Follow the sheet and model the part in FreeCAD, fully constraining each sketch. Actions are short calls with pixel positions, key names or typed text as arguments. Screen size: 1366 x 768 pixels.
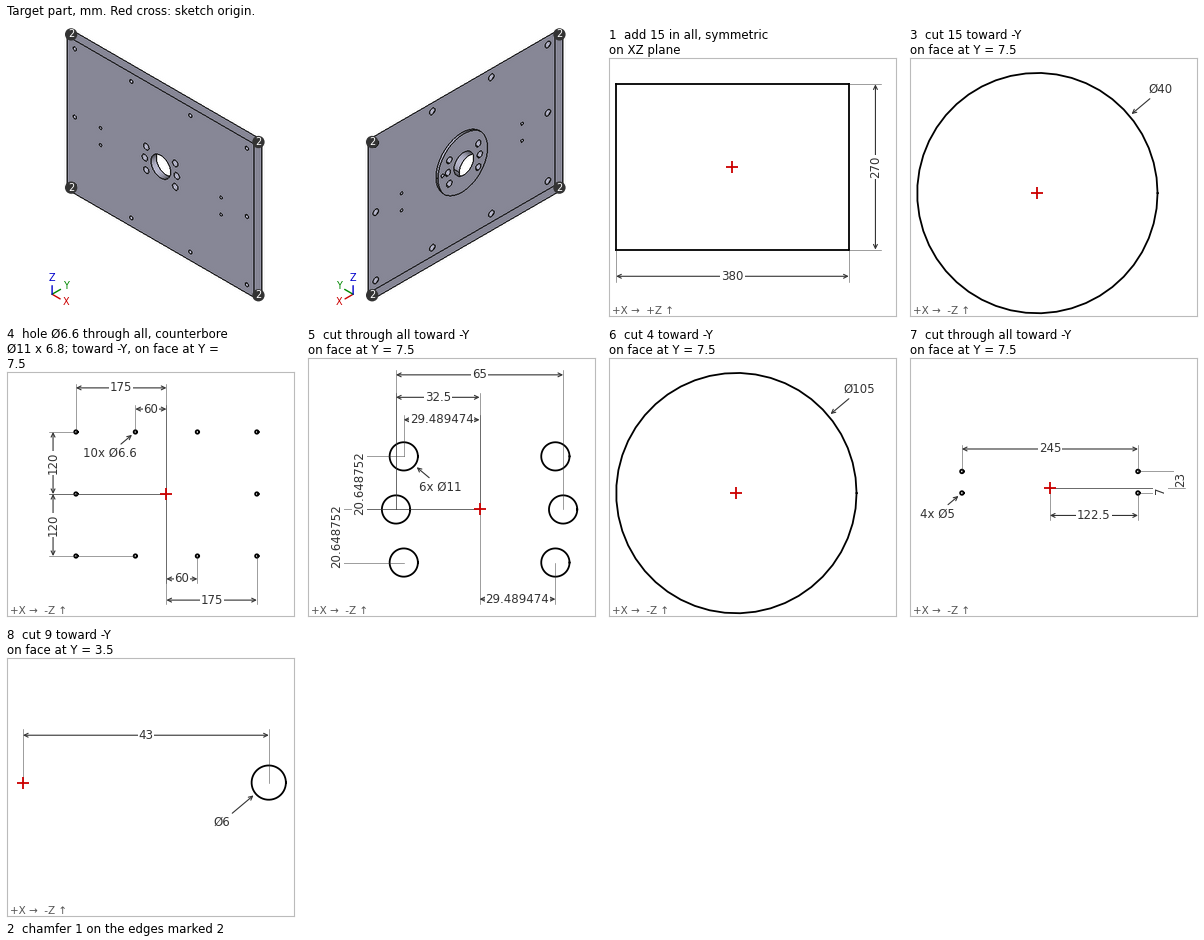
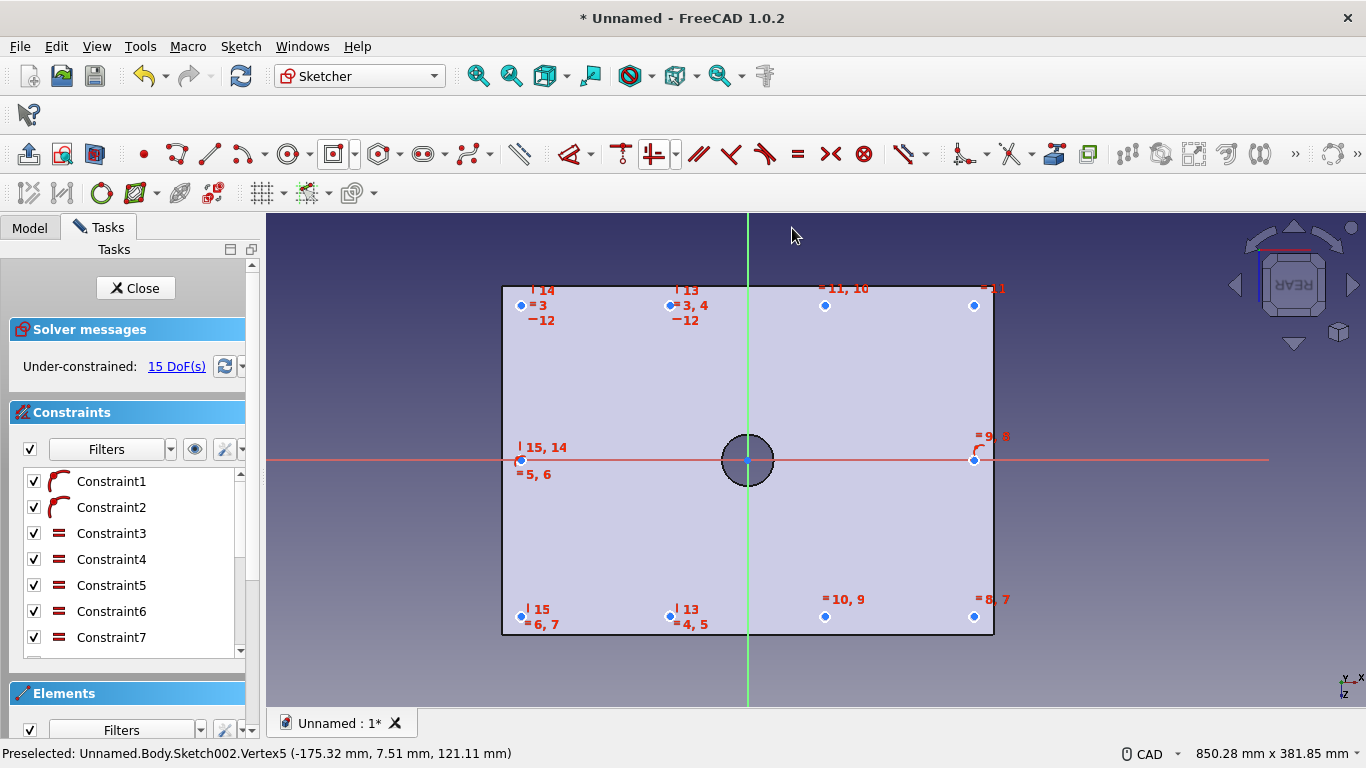
click(670, 616)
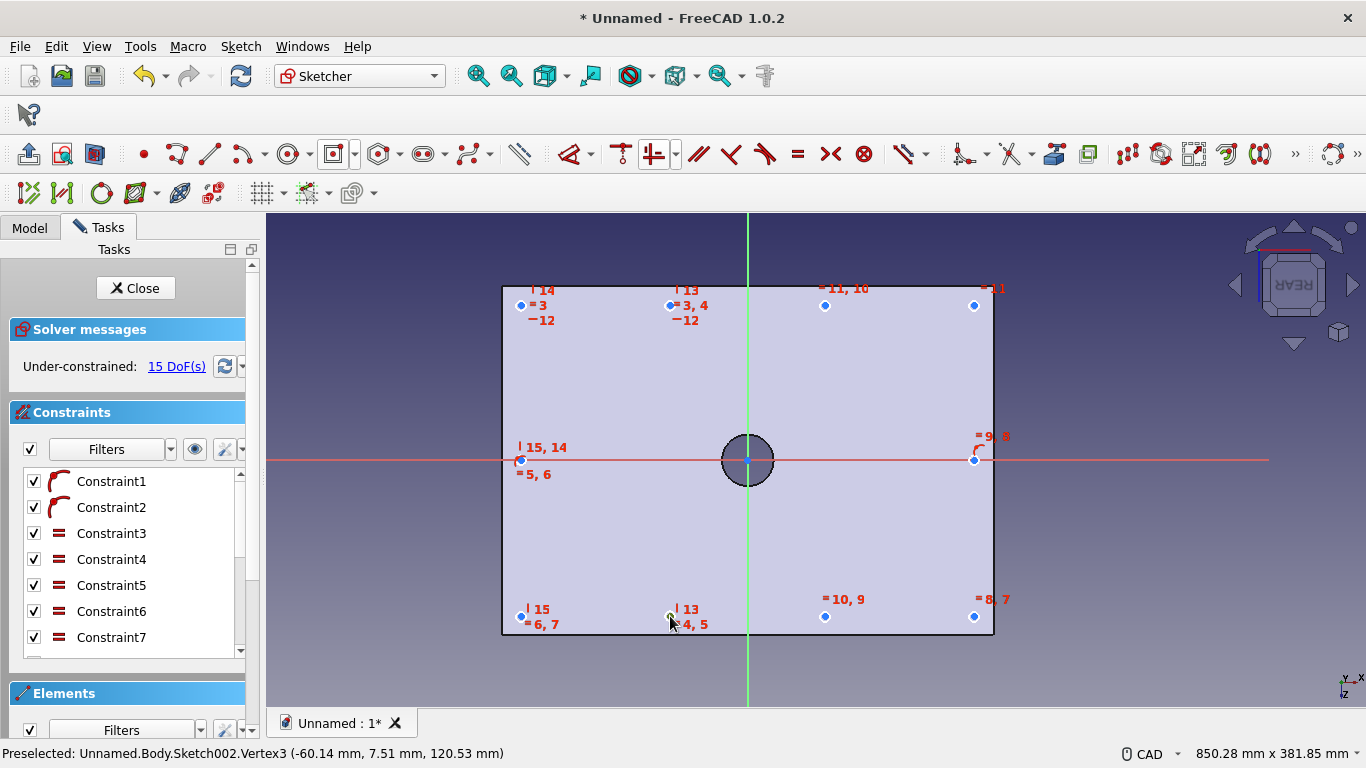
click(521, 617)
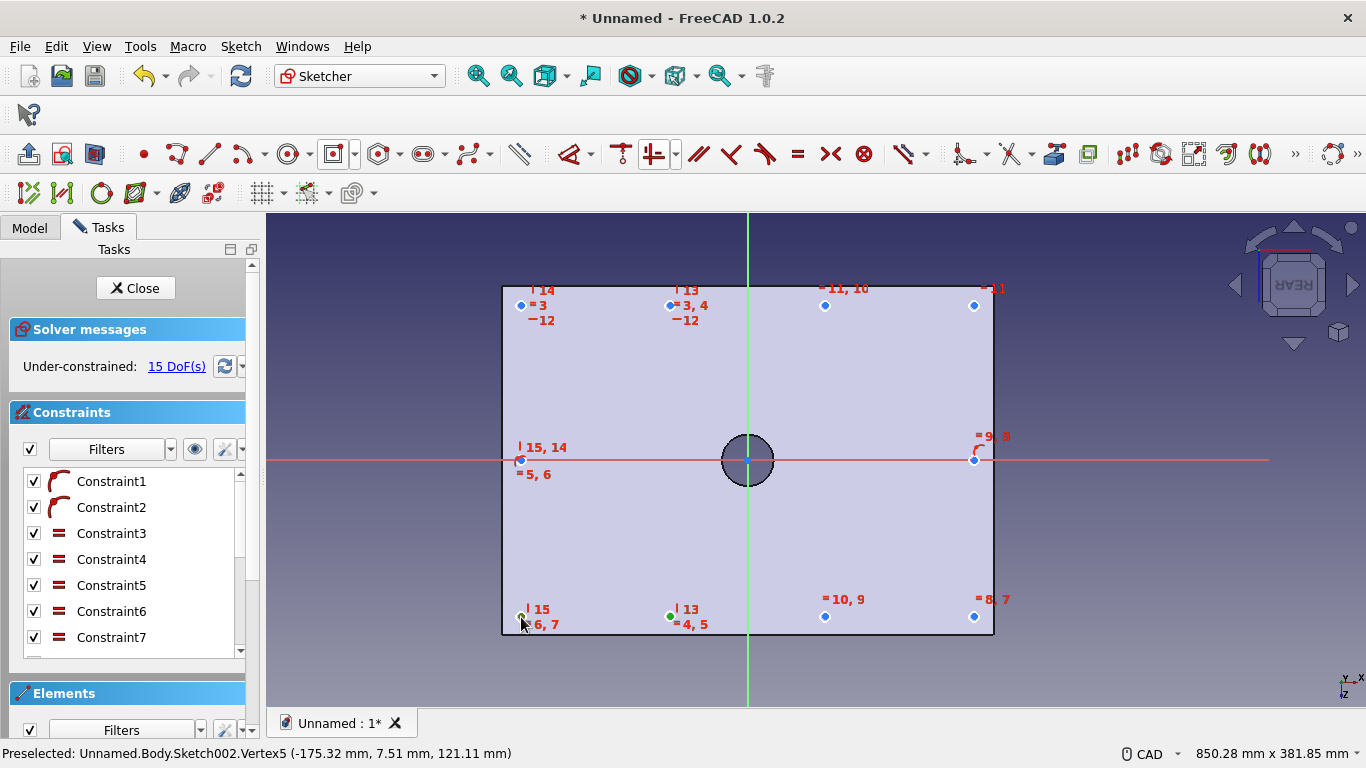
click(676, 154)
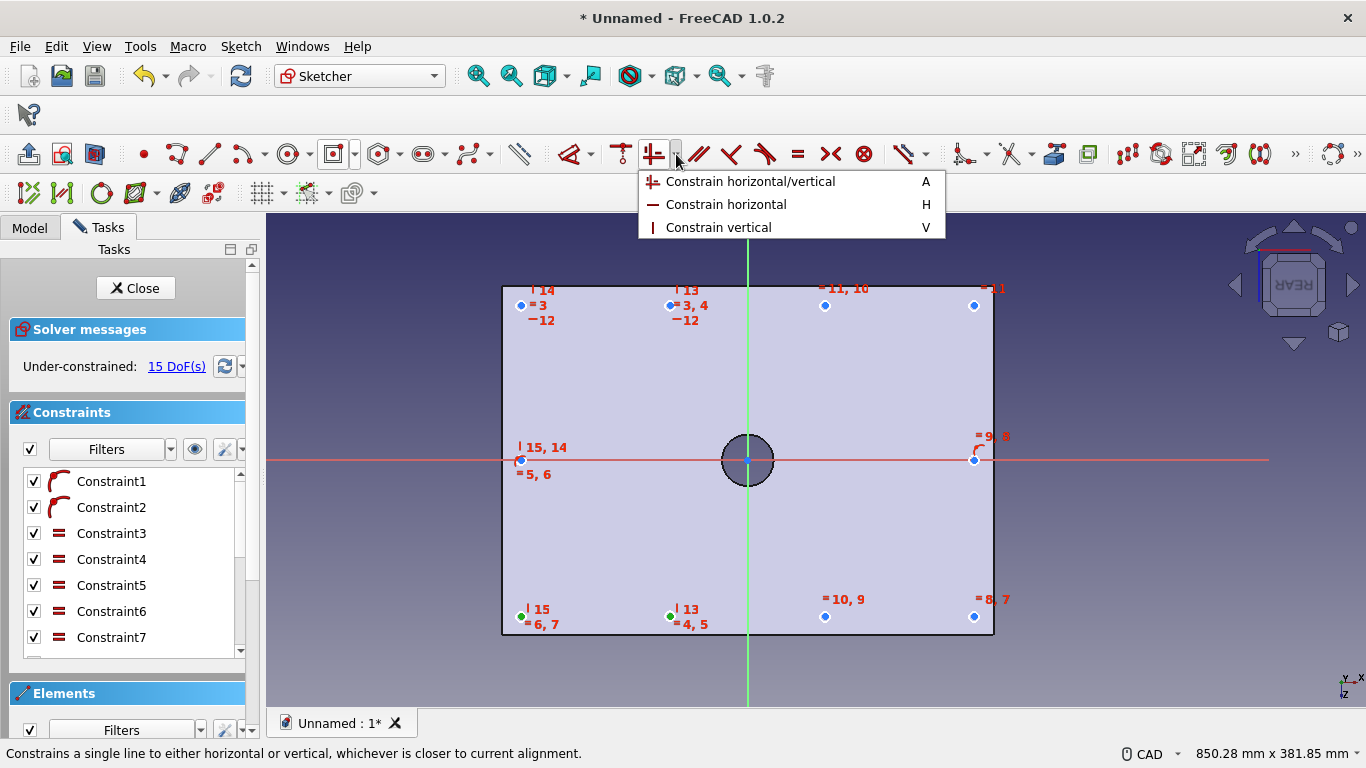
click(792, 204)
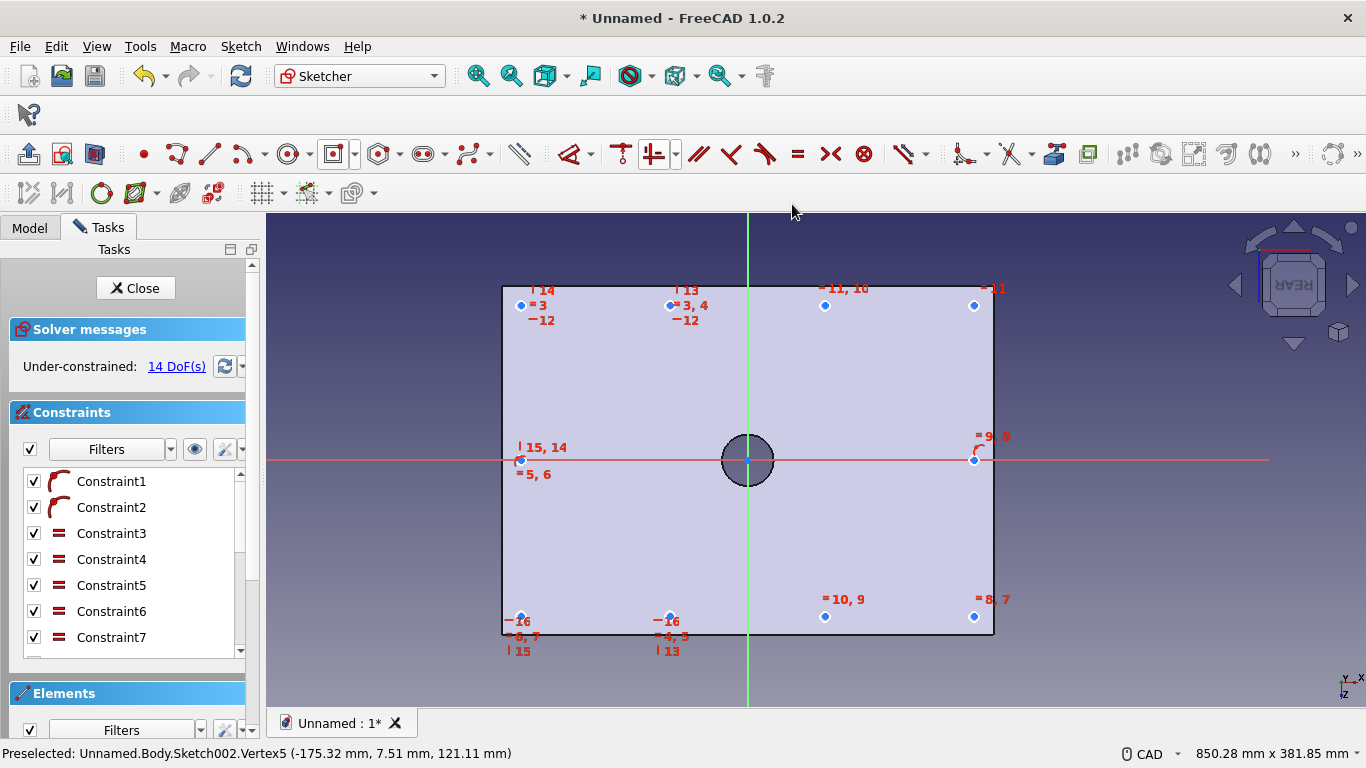
click(670, 616)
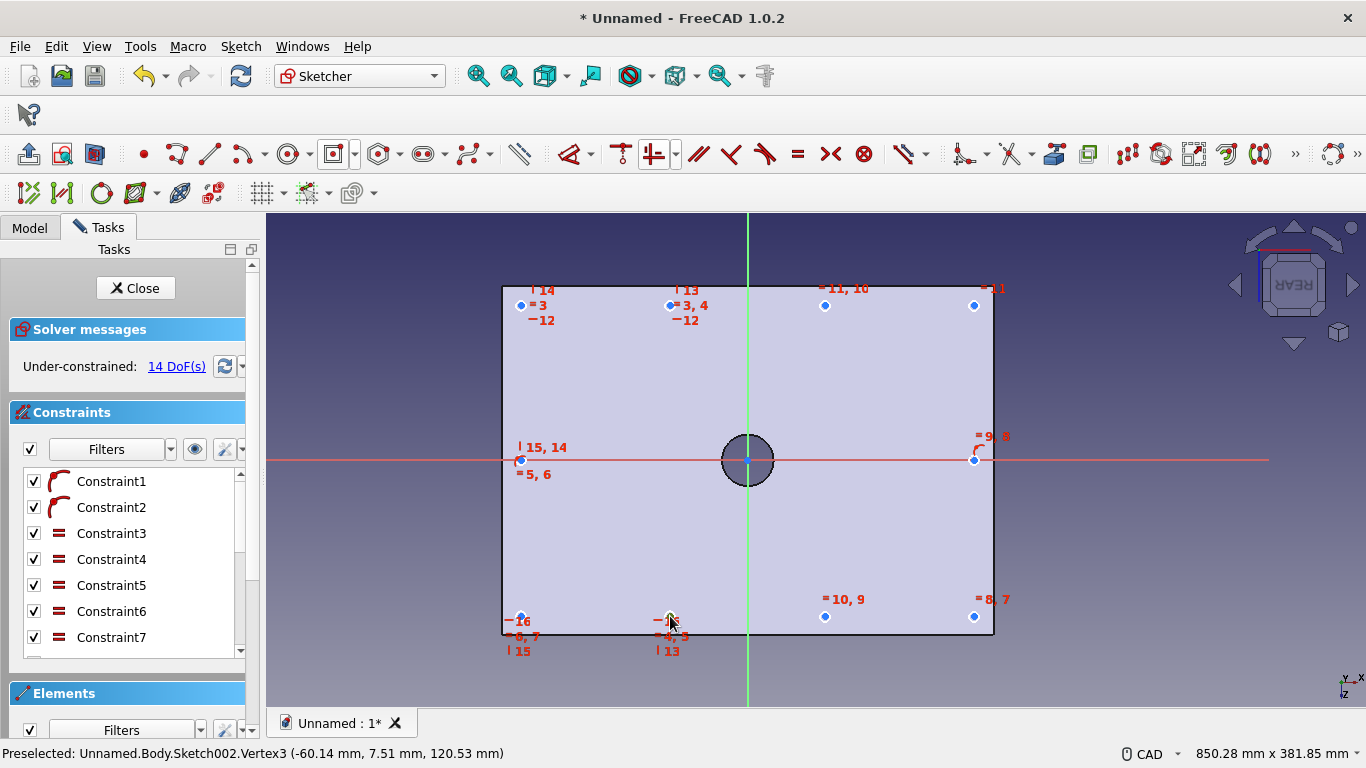
click(974, 617)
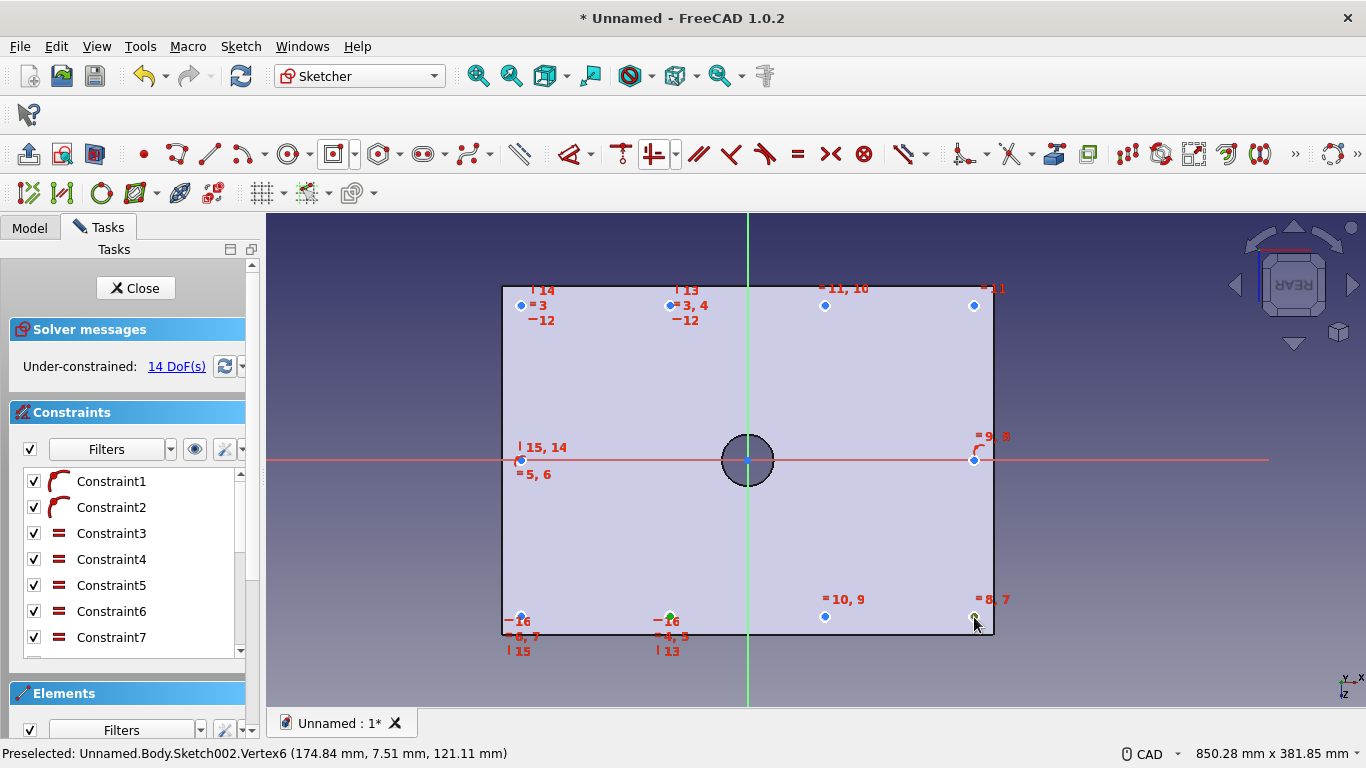
key(h)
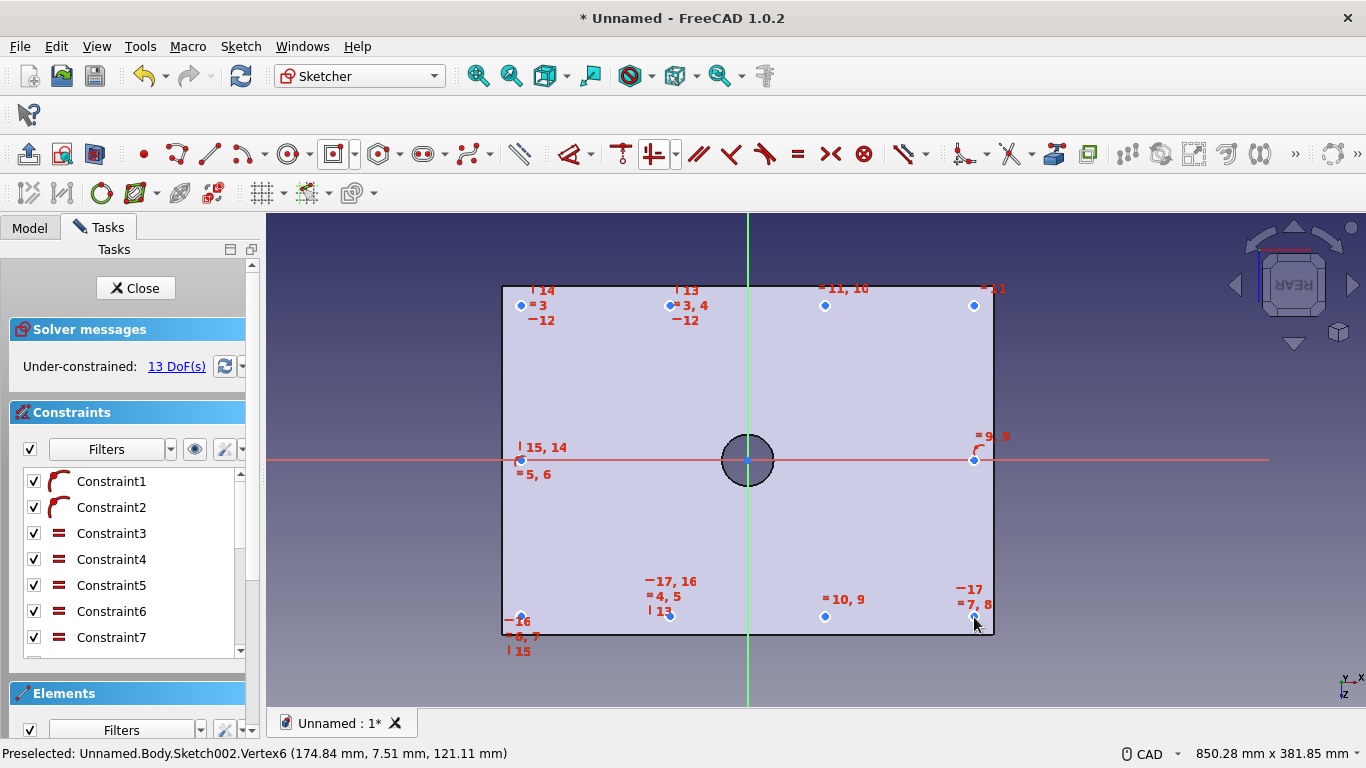
click(974, 616)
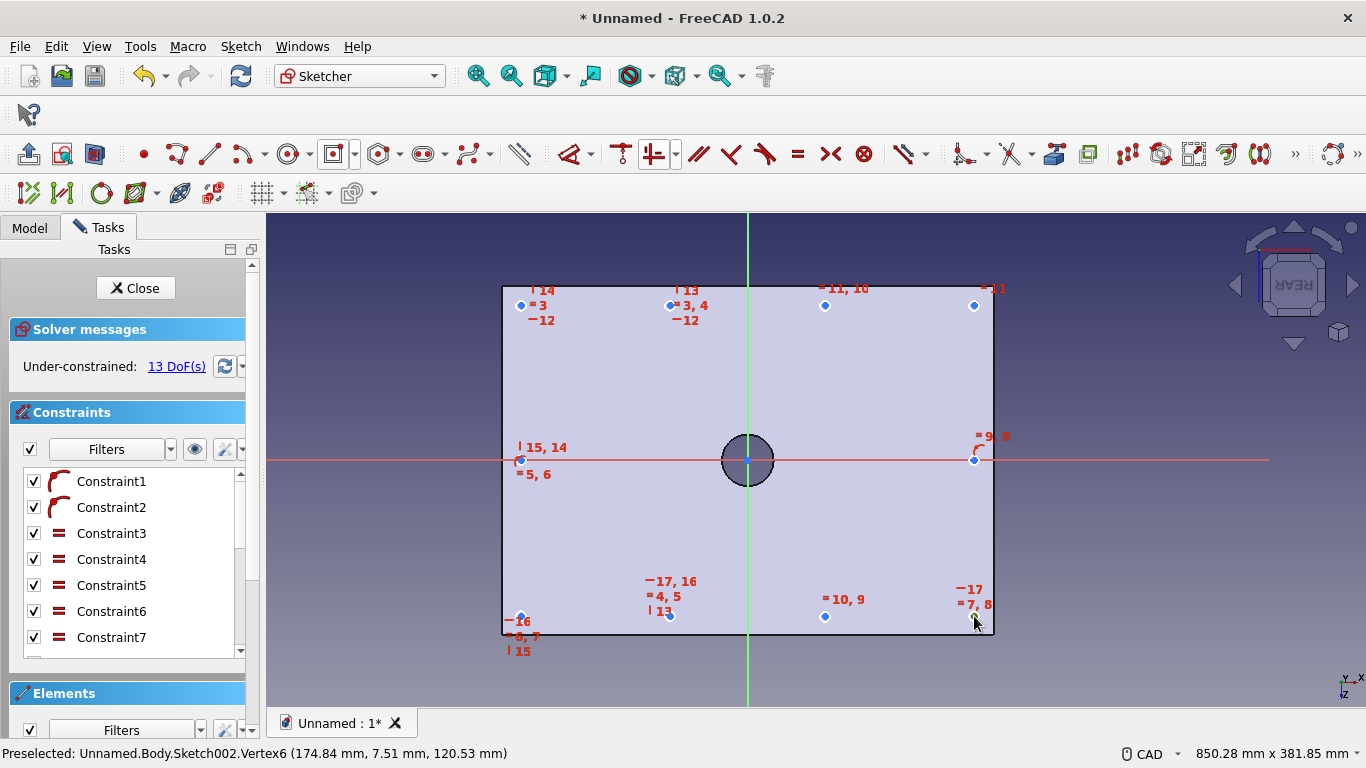
click(974, 460)